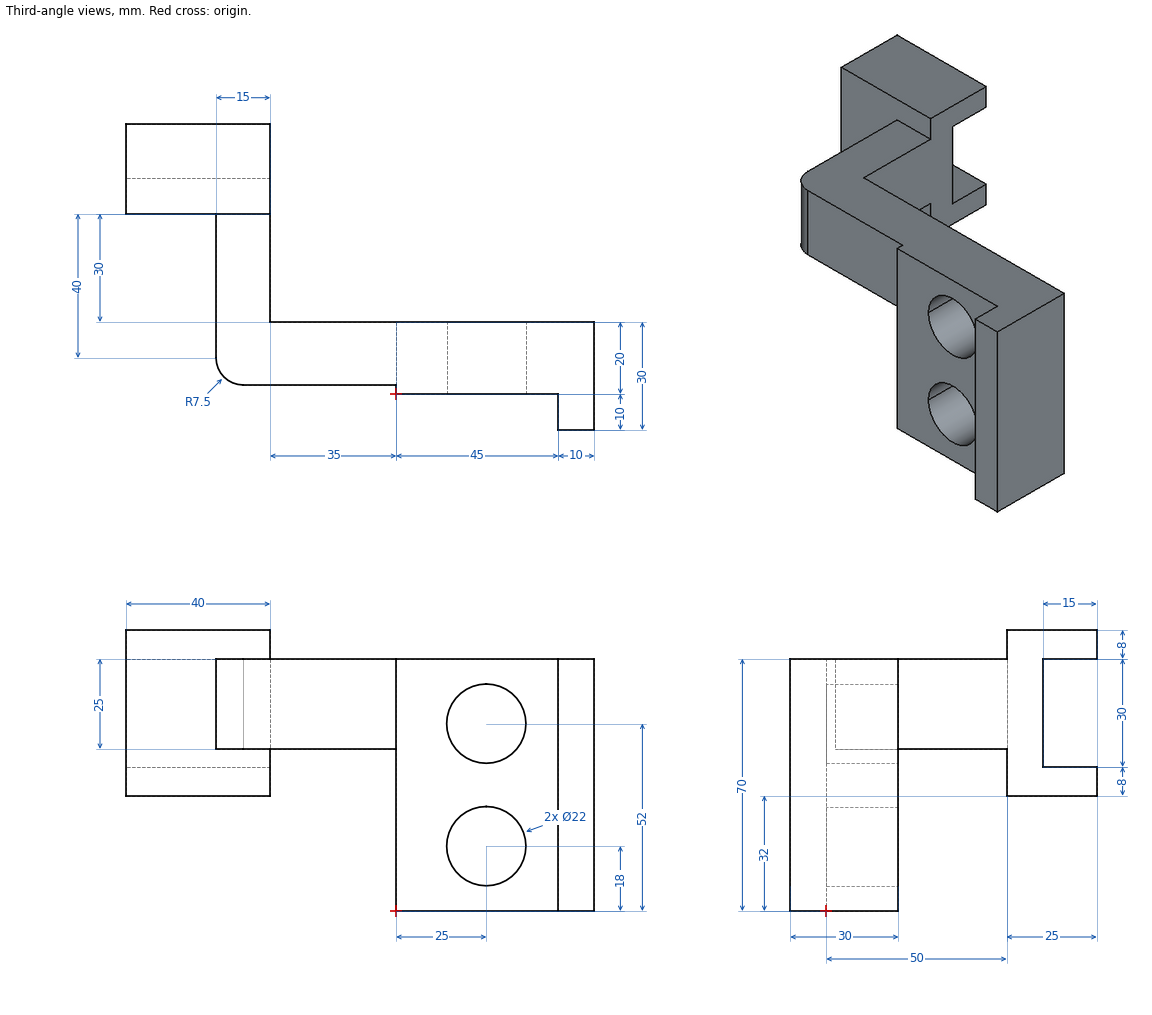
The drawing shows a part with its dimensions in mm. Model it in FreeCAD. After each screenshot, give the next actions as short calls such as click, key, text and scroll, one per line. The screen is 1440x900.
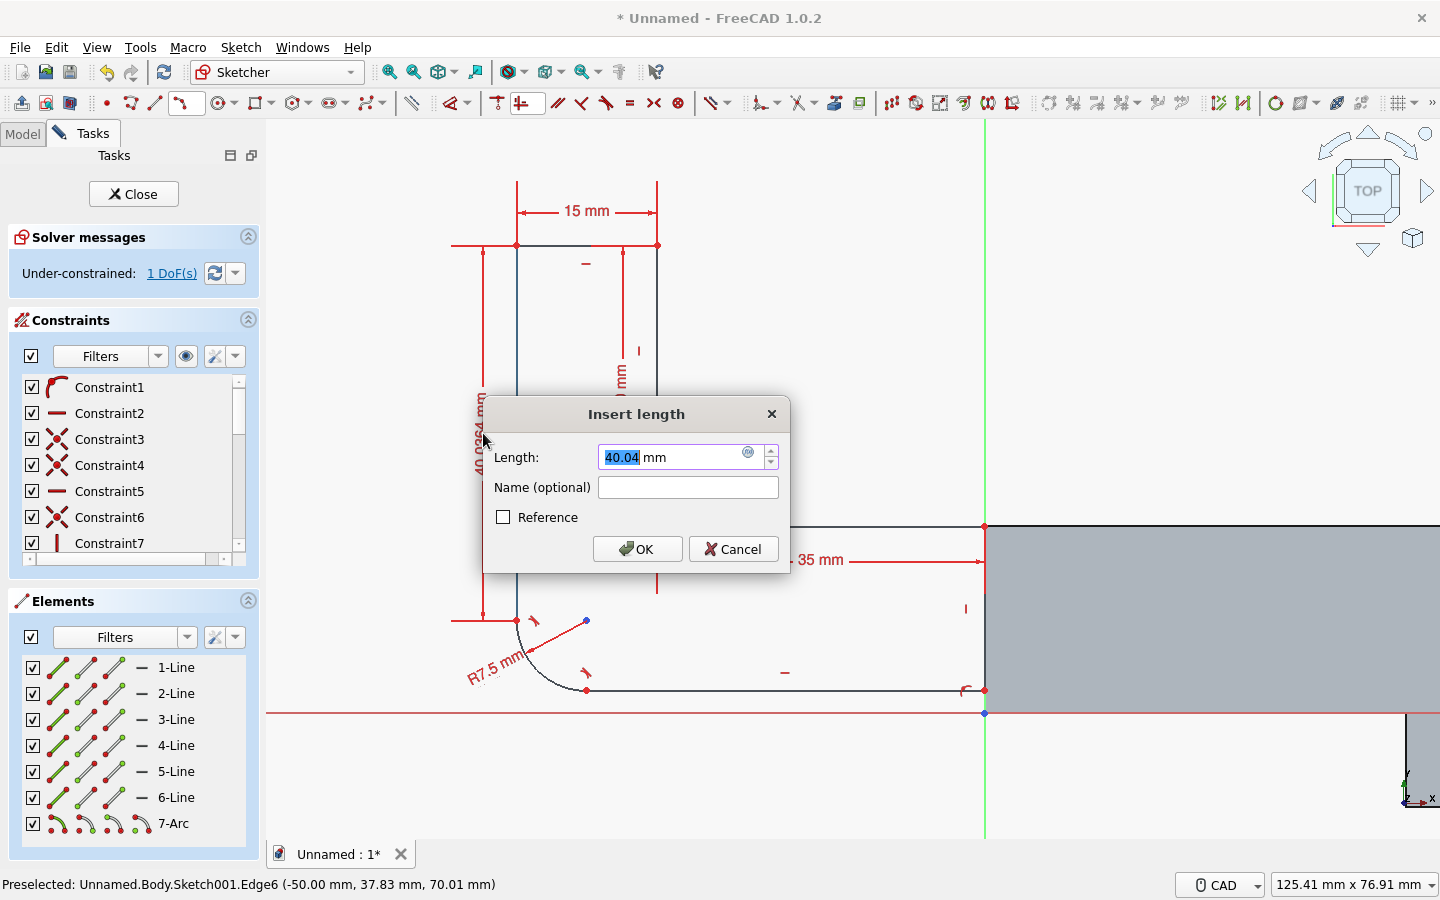
text(40)
key(Return)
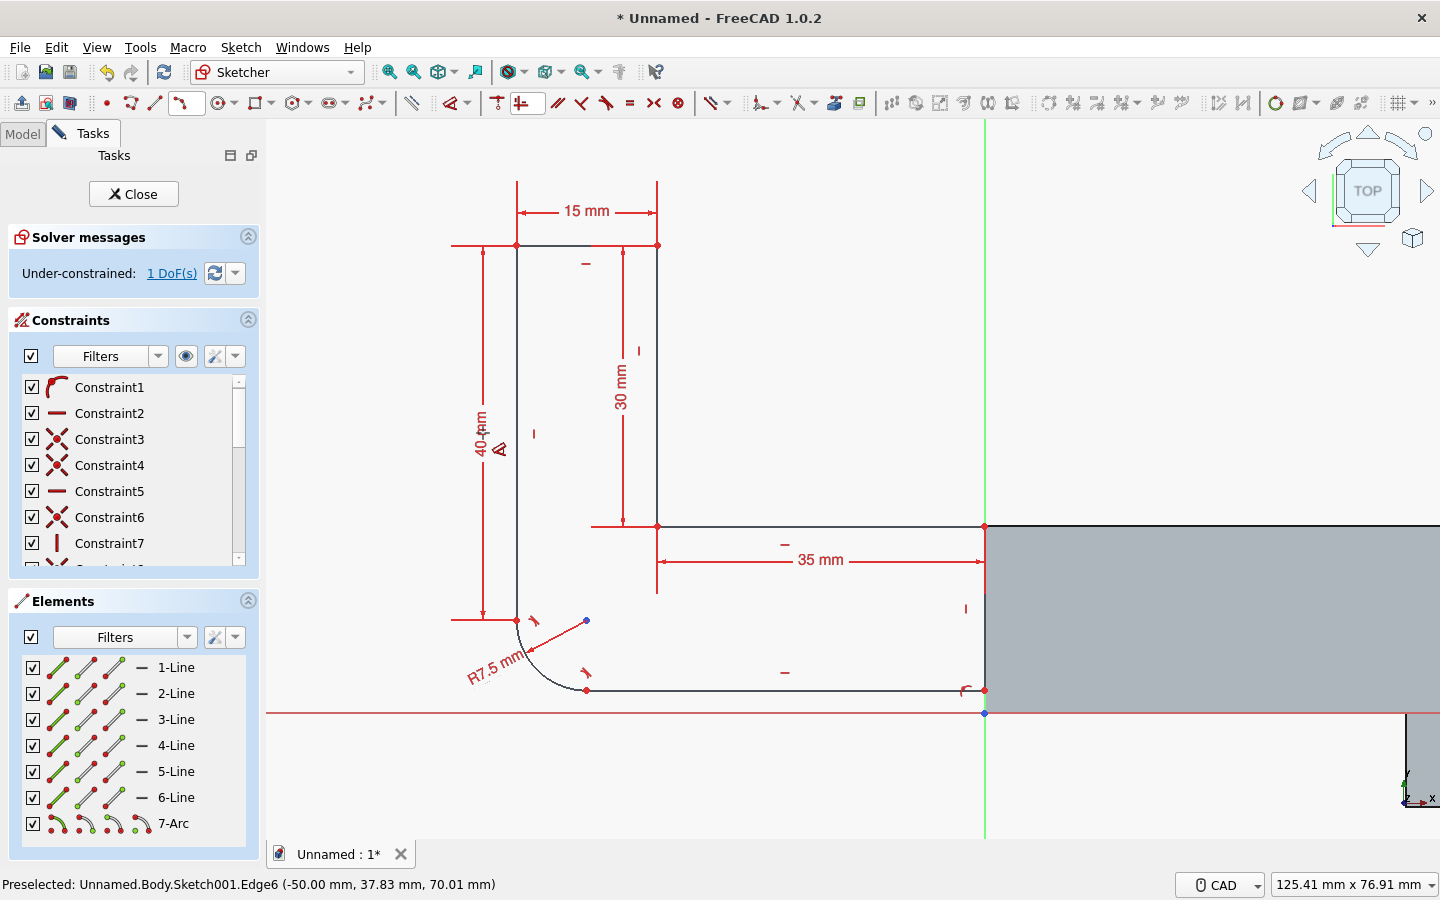
click(985, 527)
click(1019, 620)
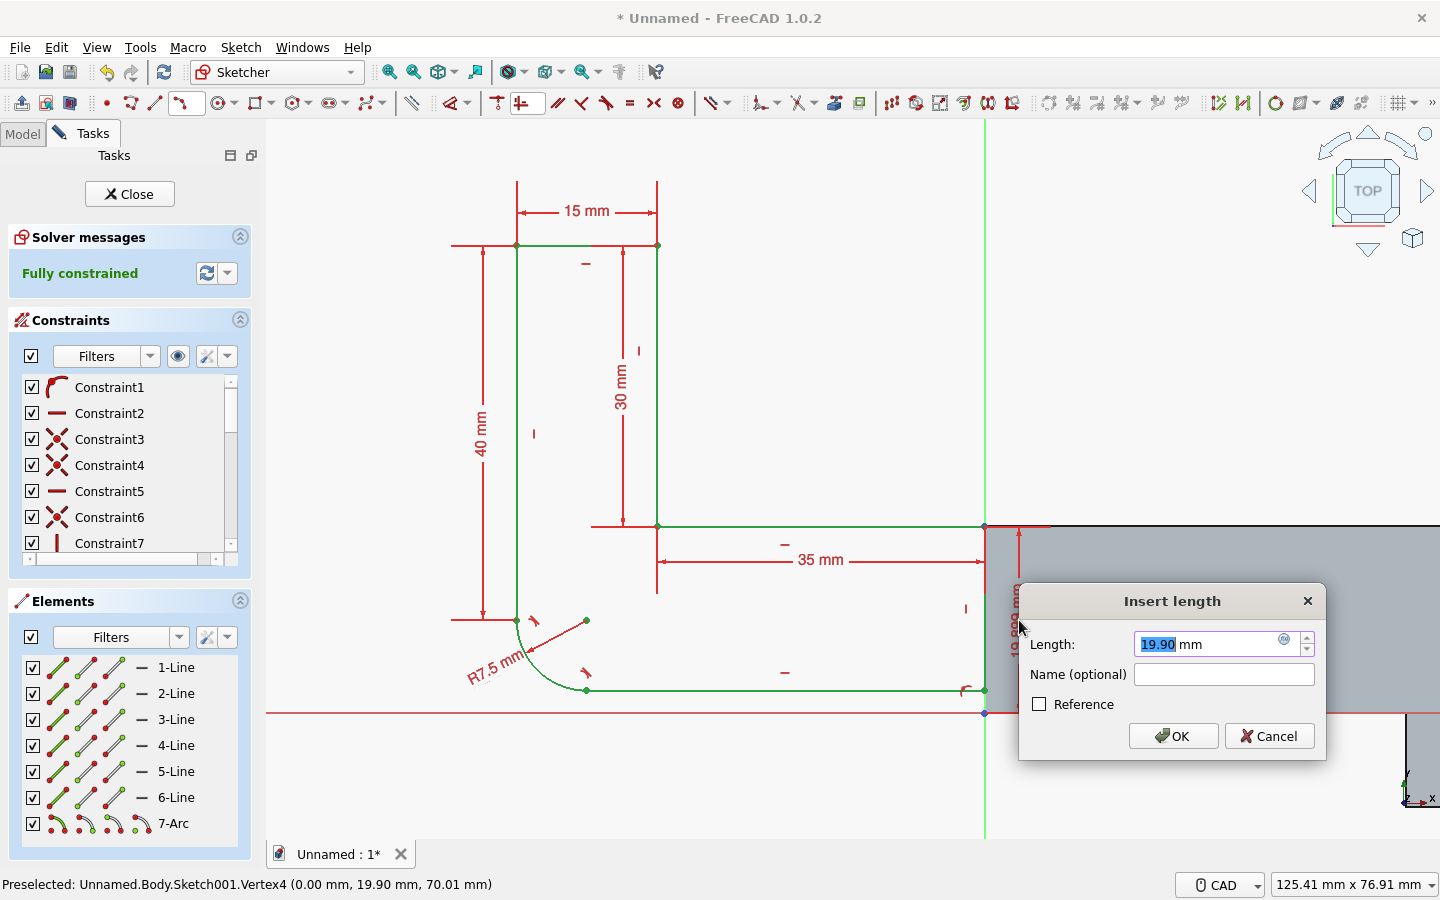
text(20)
key(Return)
key(Escape)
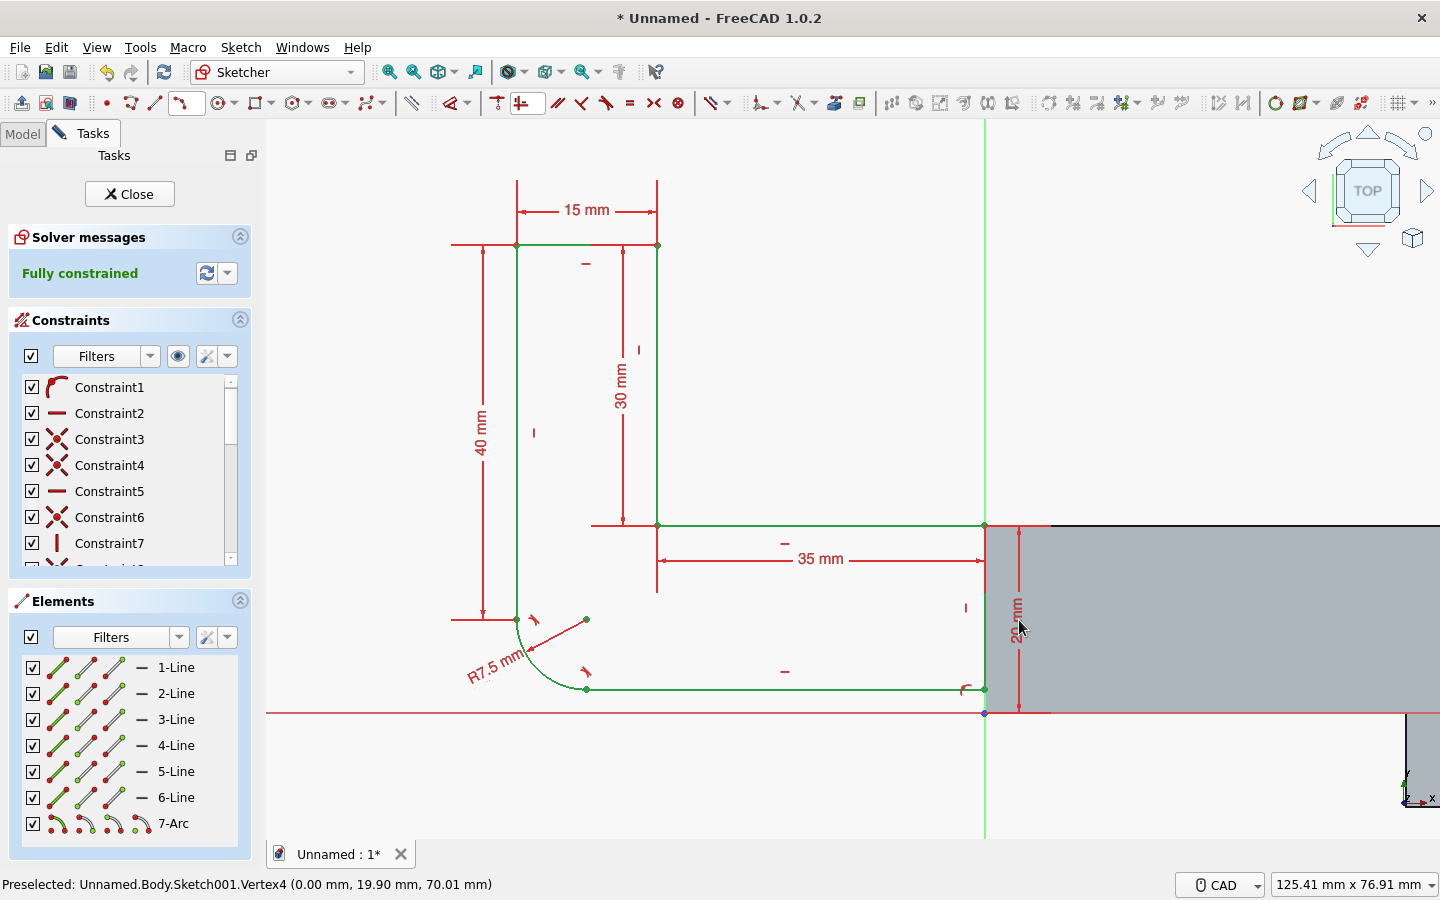
click(130, 194)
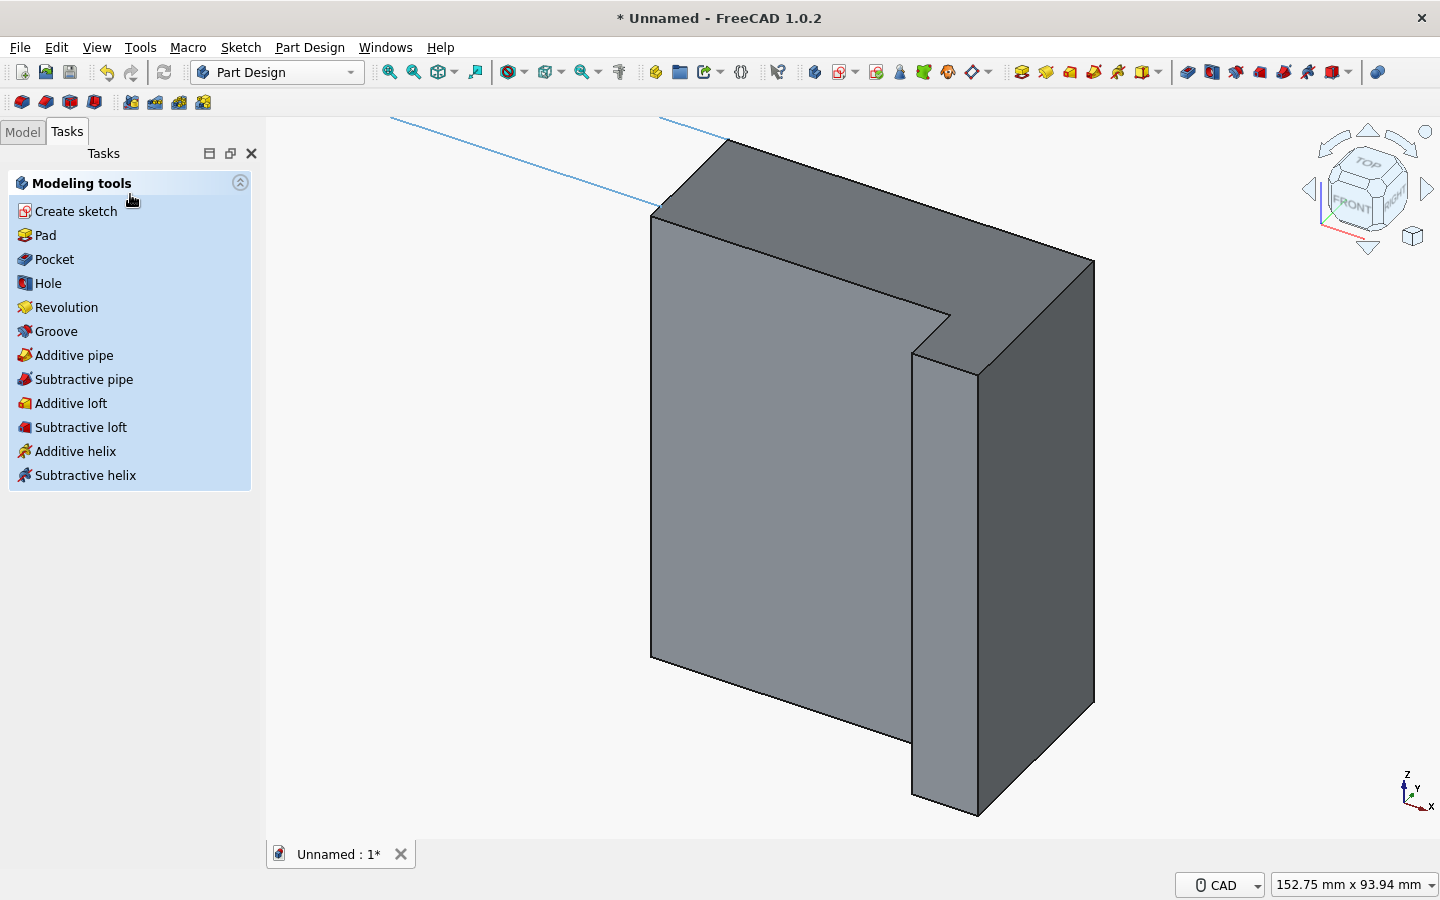
click(1022, 72)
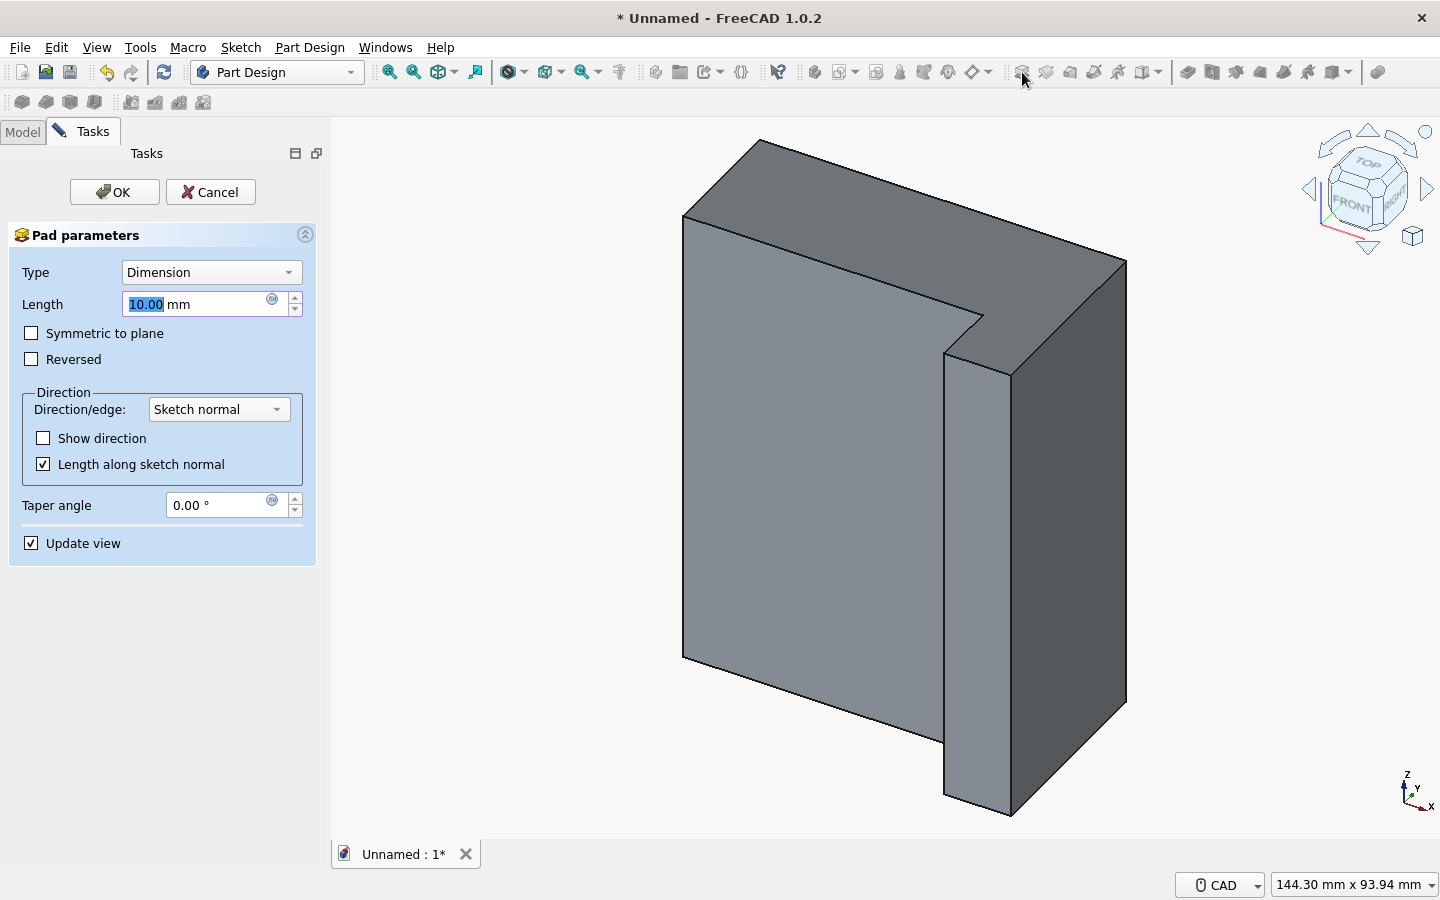
text(25)
key(Tab)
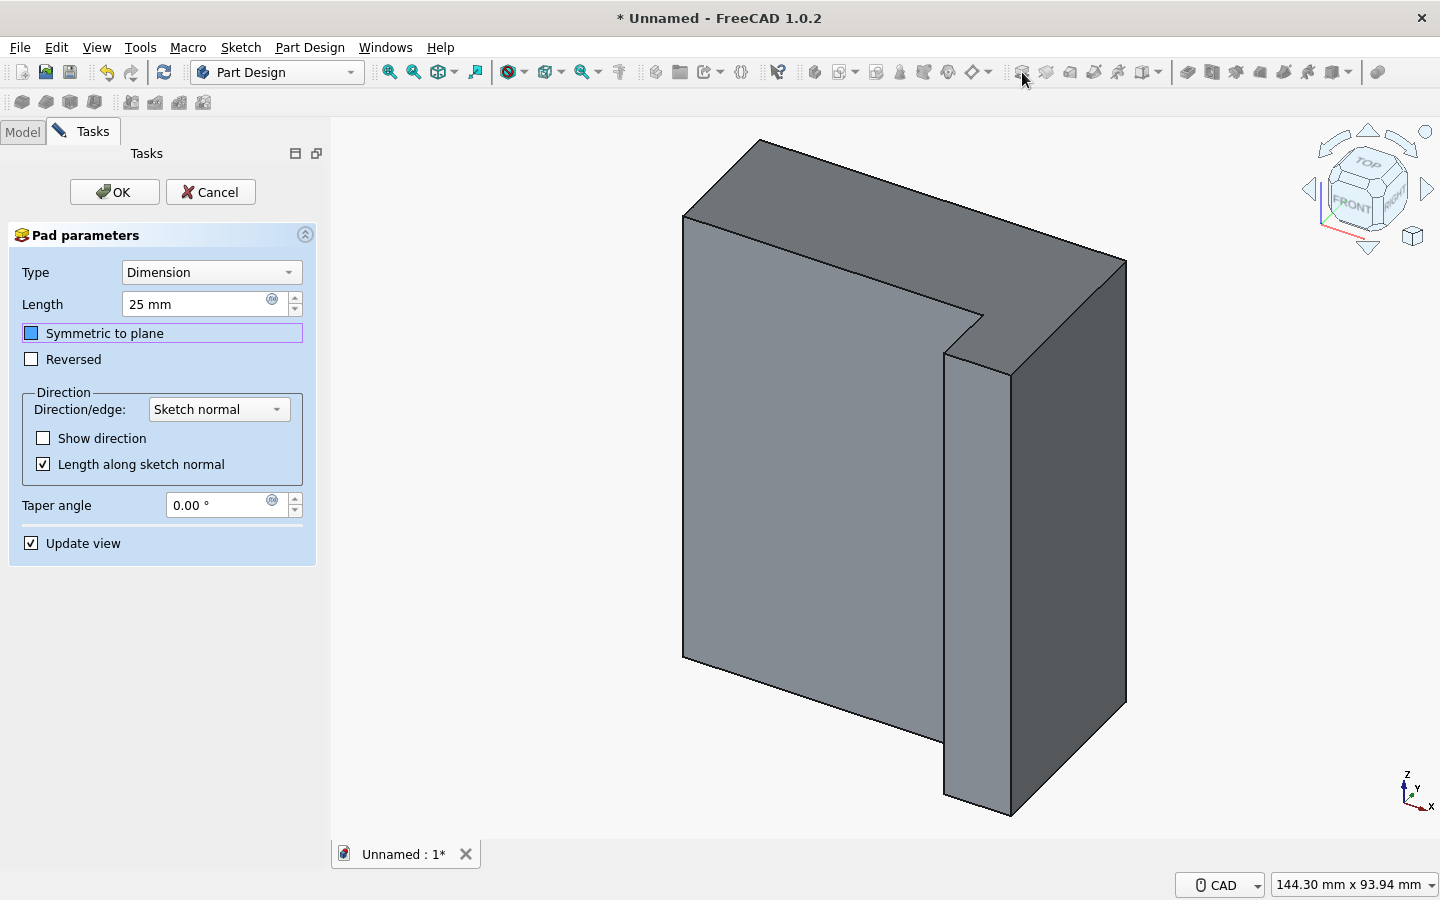
click(30, 359)